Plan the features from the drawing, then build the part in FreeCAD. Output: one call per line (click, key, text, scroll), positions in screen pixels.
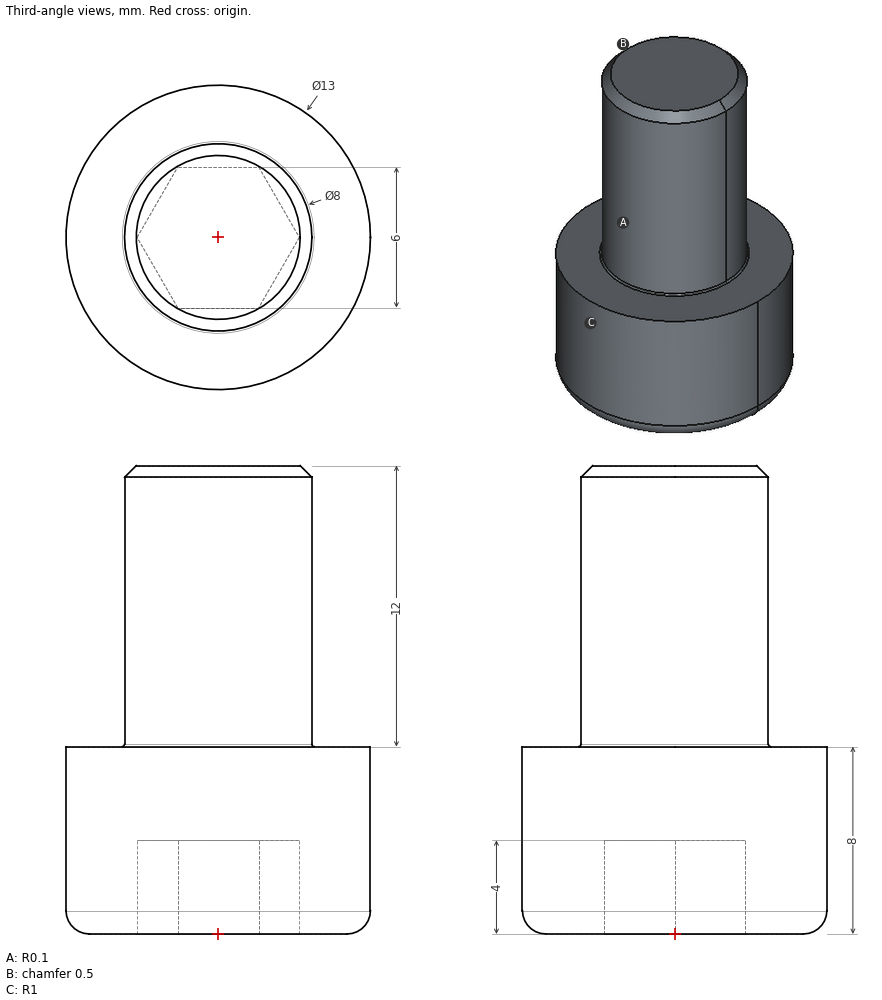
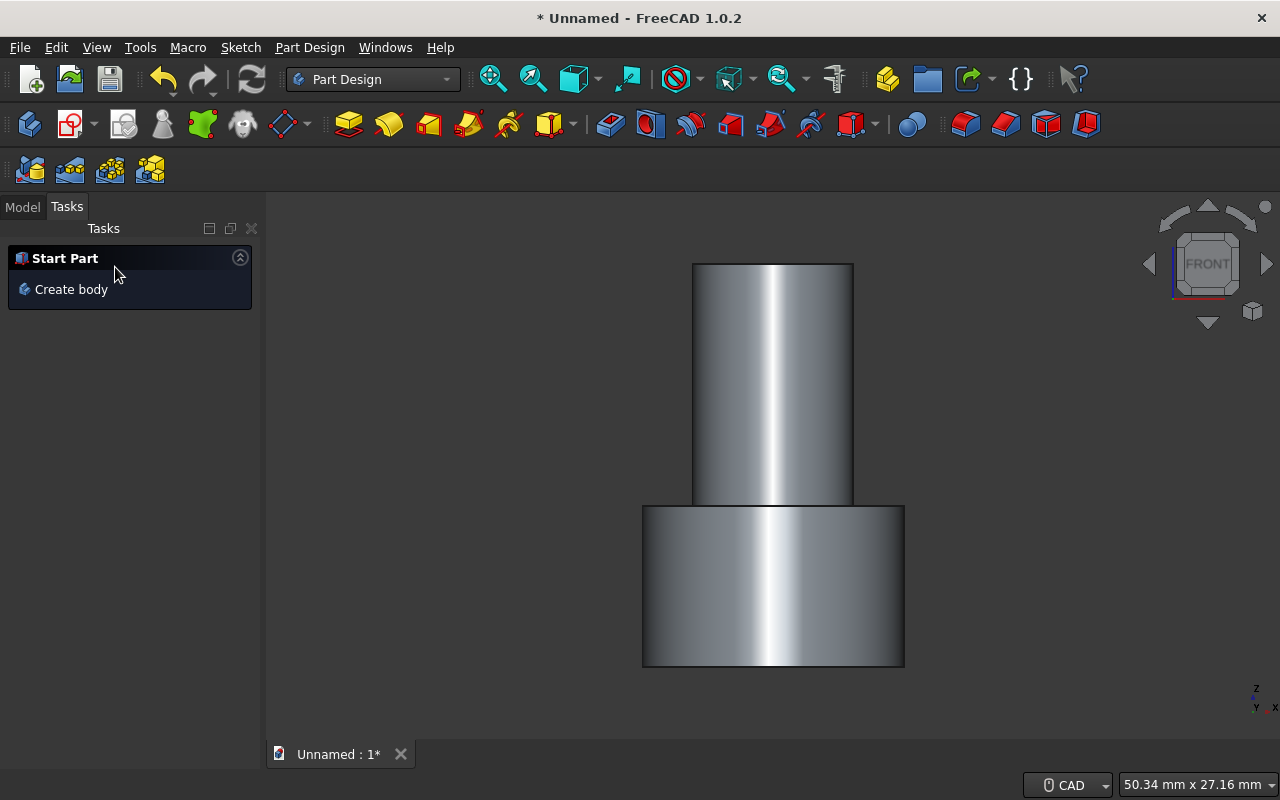
key(3)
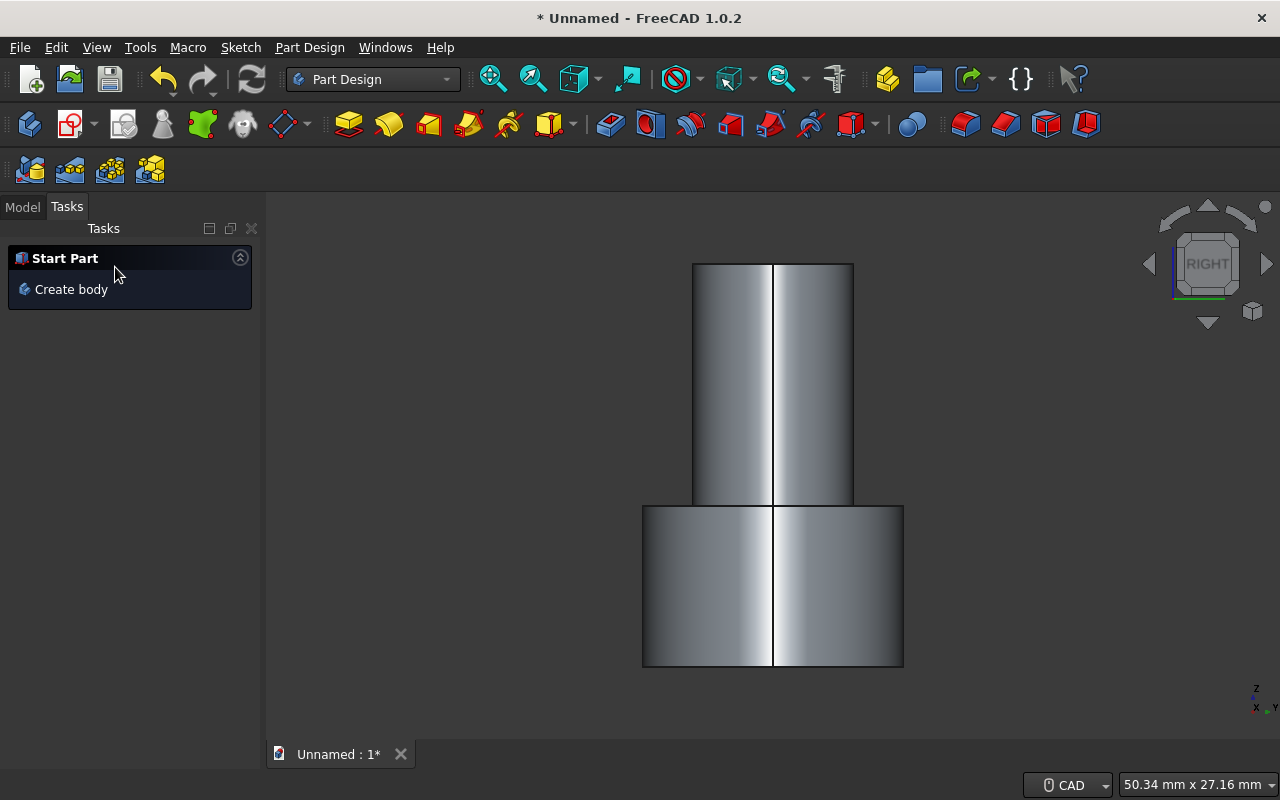
key(5)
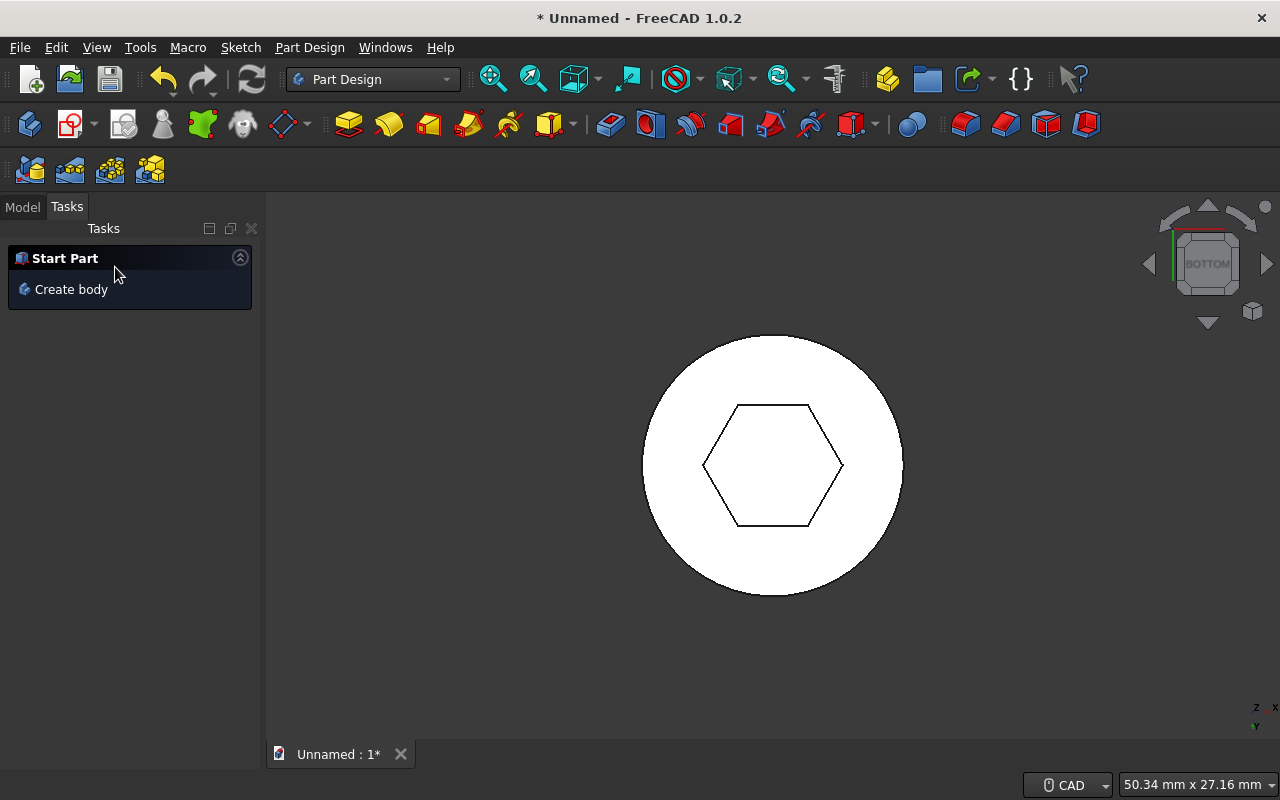
key(4)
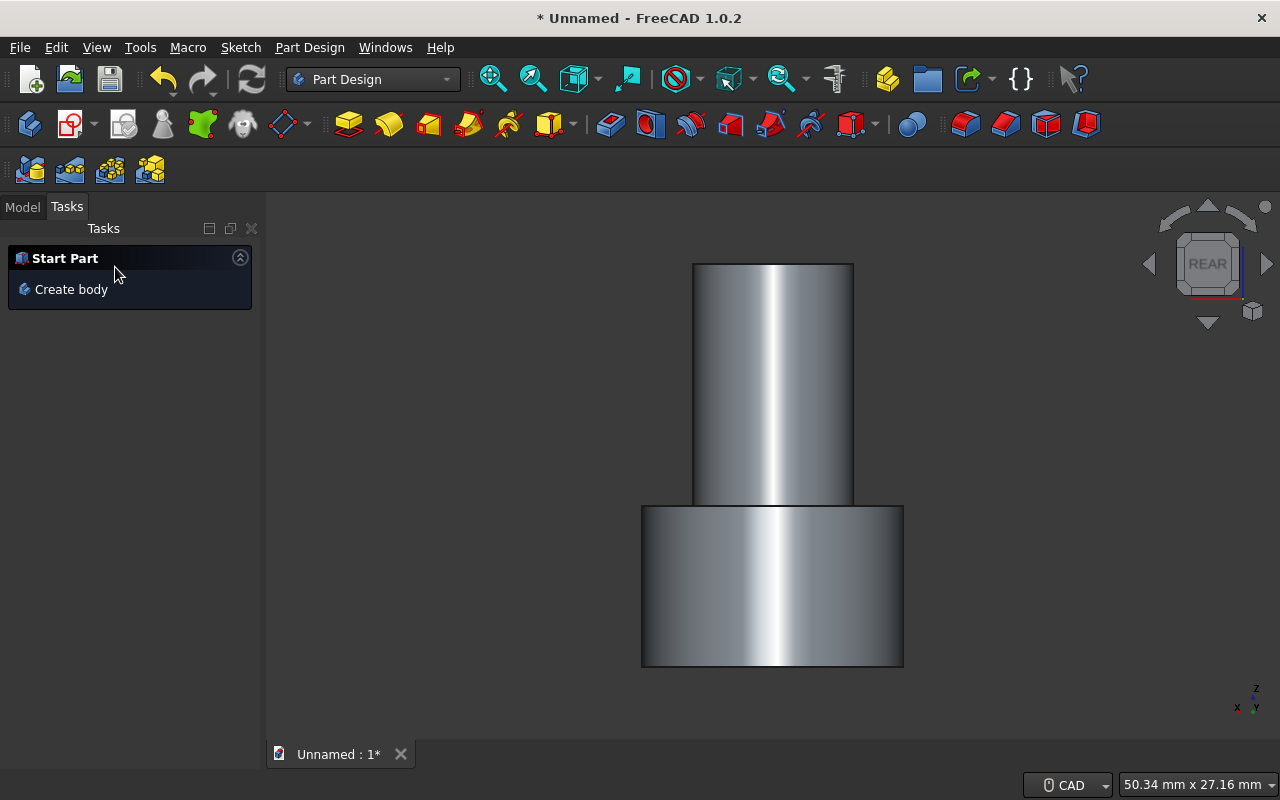
key(6)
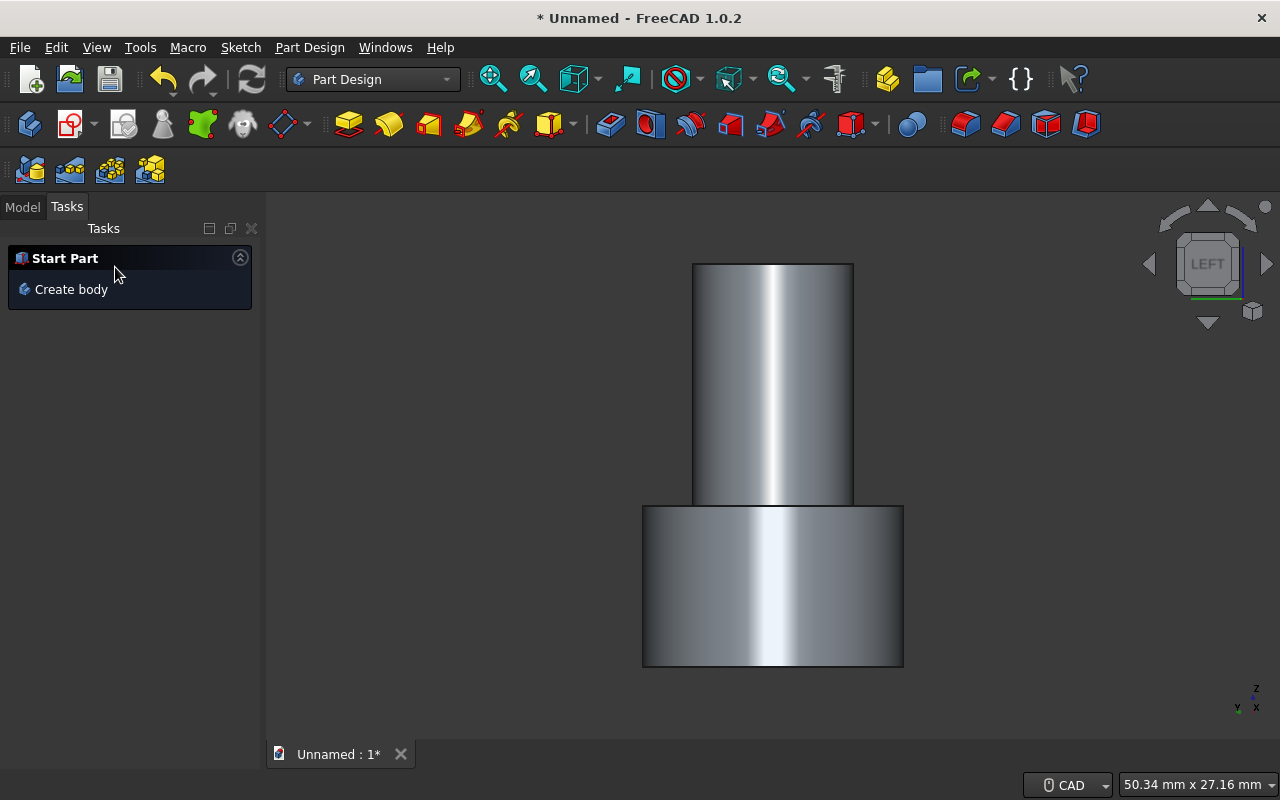
key(v)
key(3)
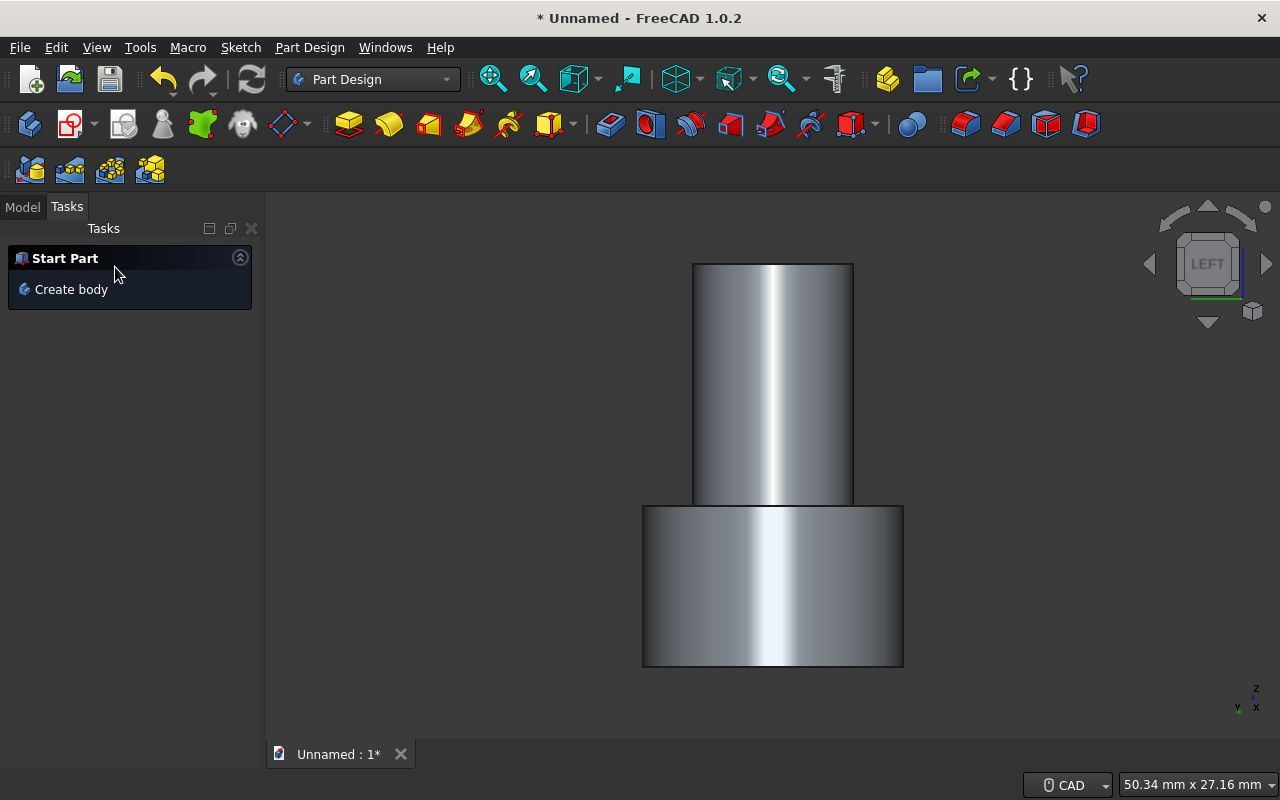
key(0)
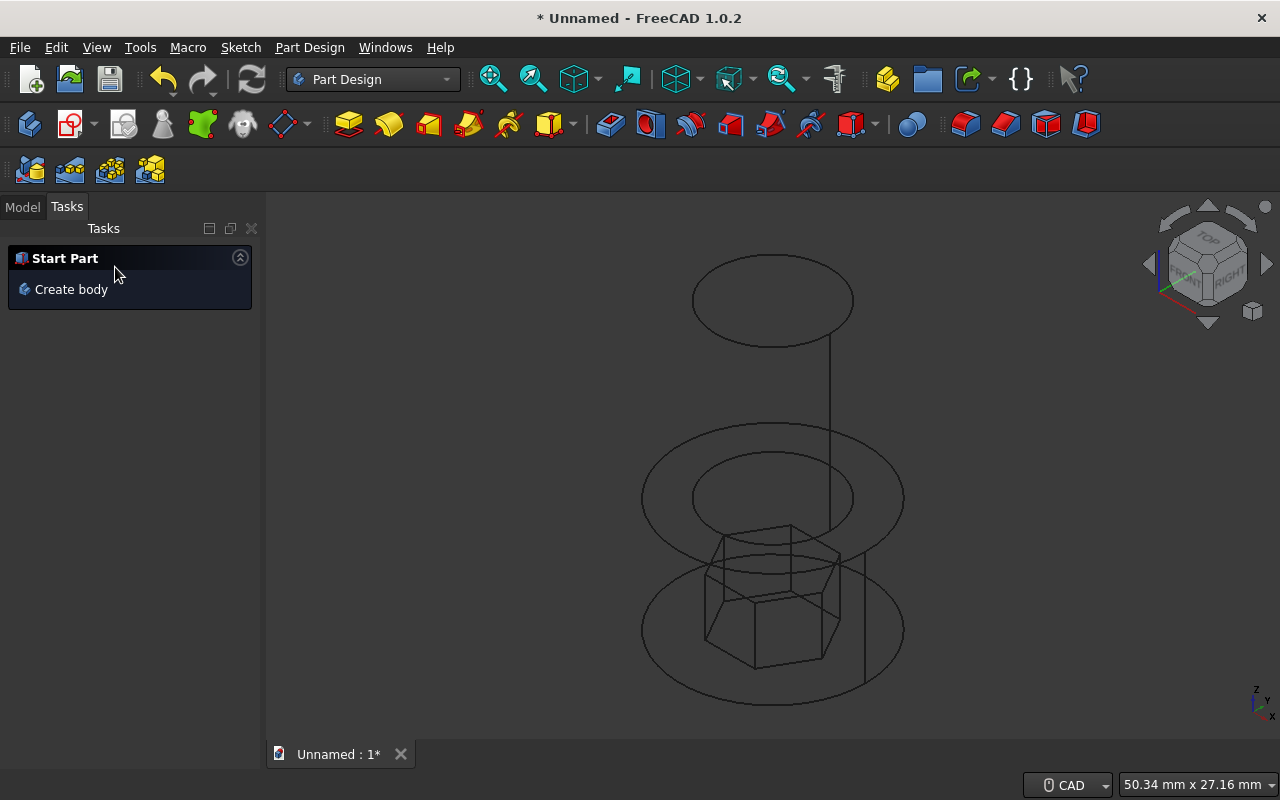
click(716, 464)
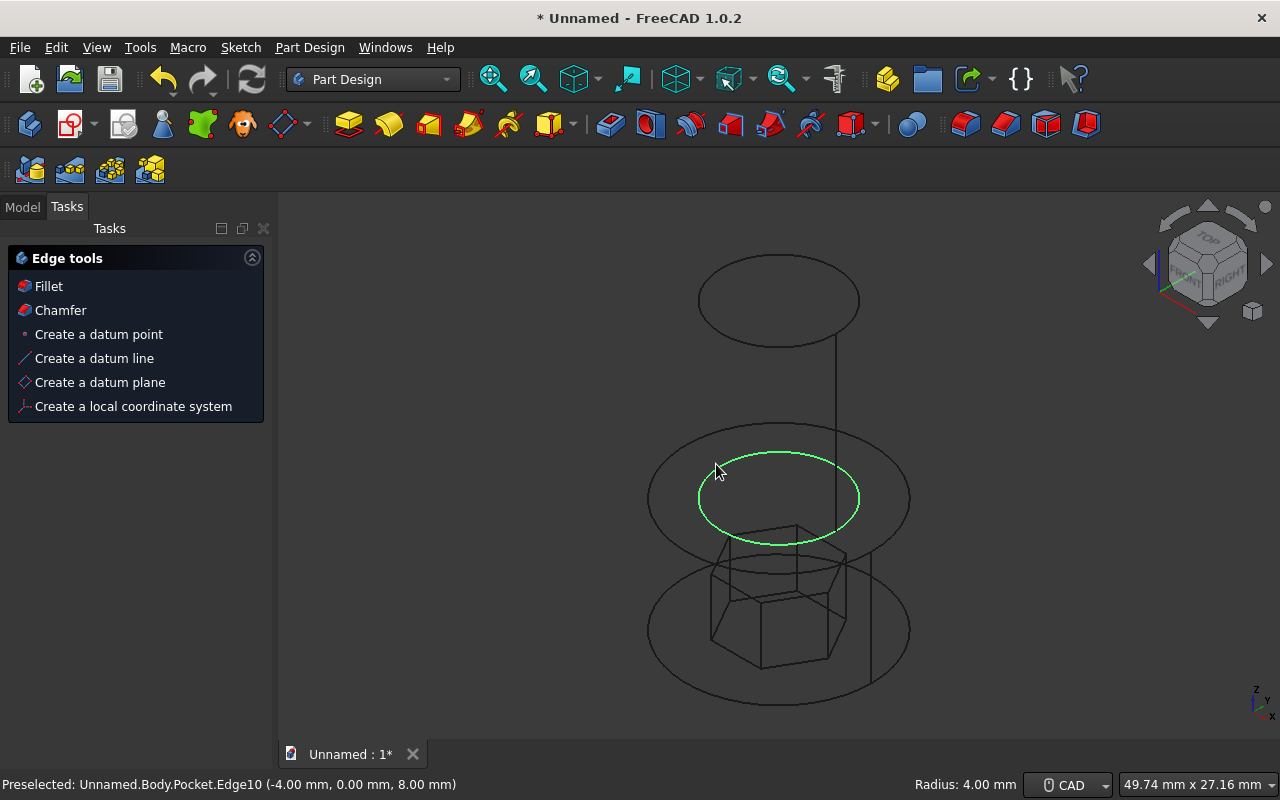
key(v)
key(1)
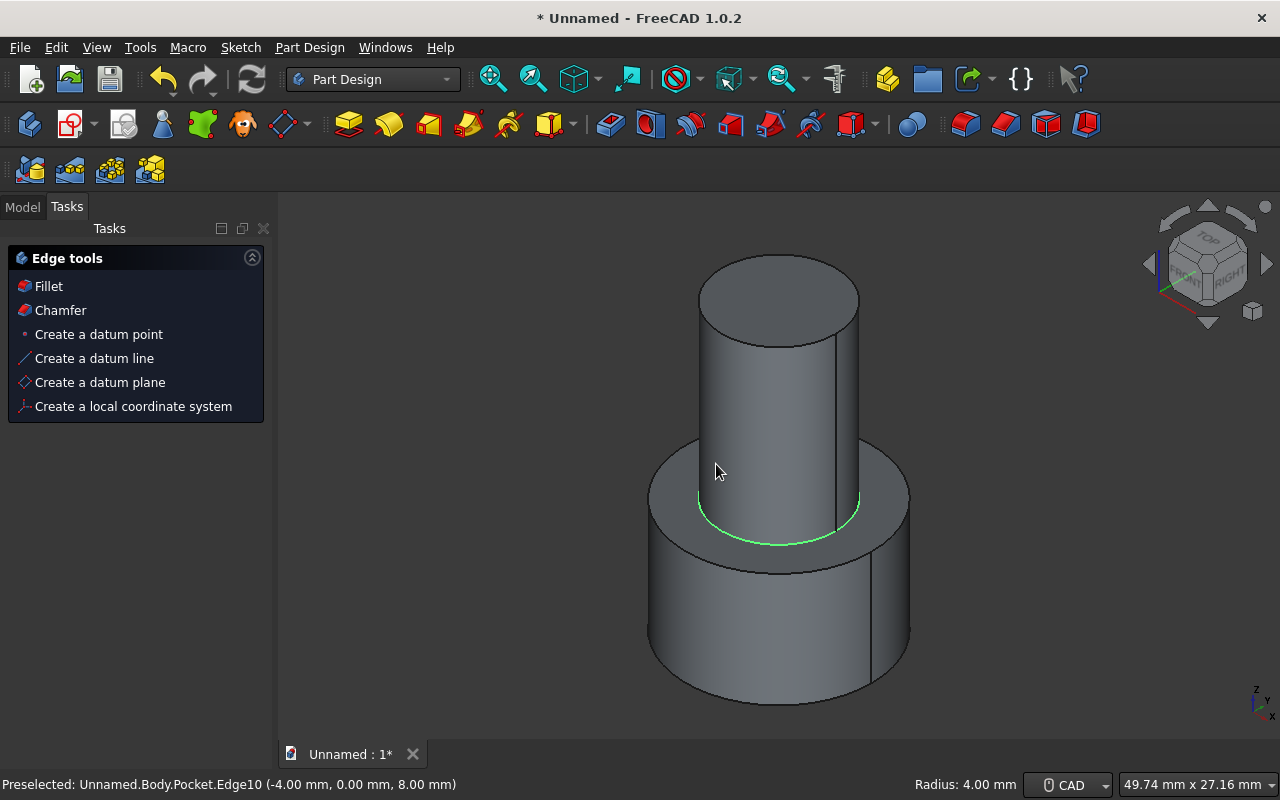
click(966, 124)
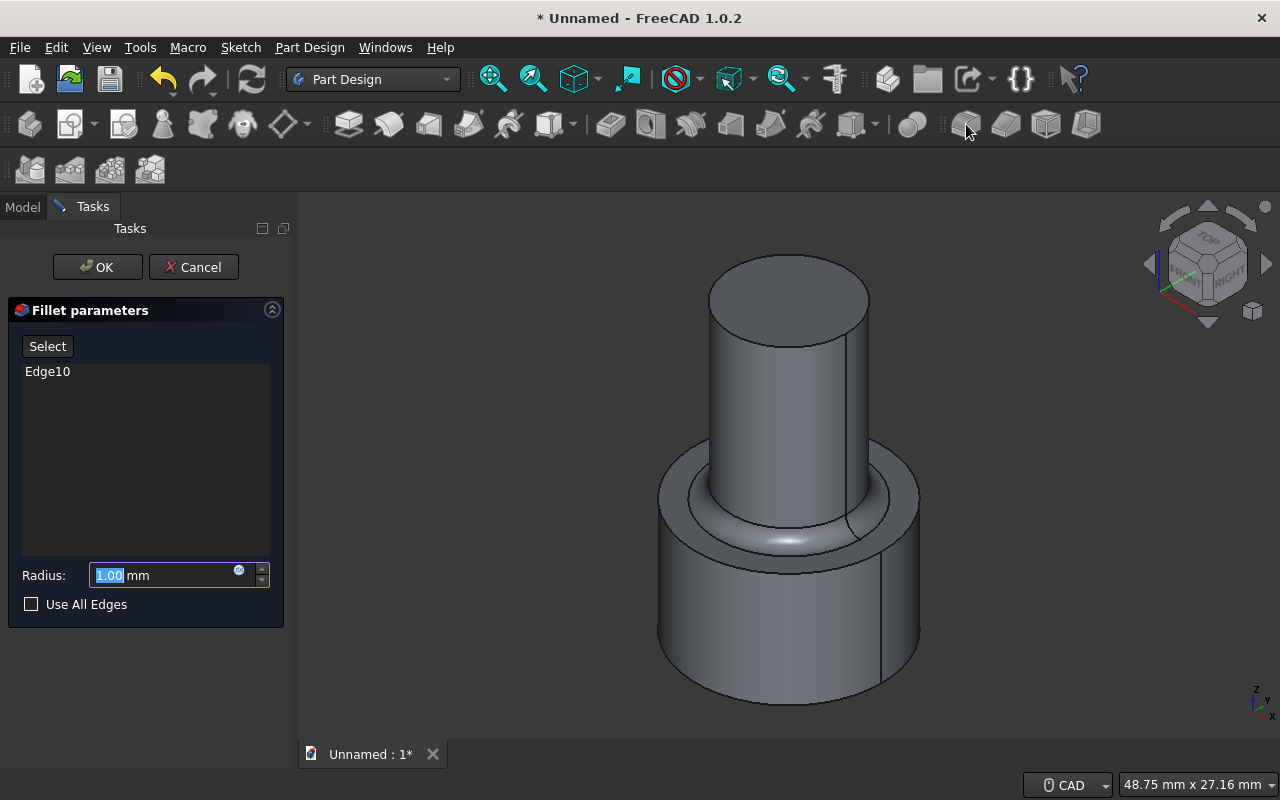
text(0.1)
key(Tab)